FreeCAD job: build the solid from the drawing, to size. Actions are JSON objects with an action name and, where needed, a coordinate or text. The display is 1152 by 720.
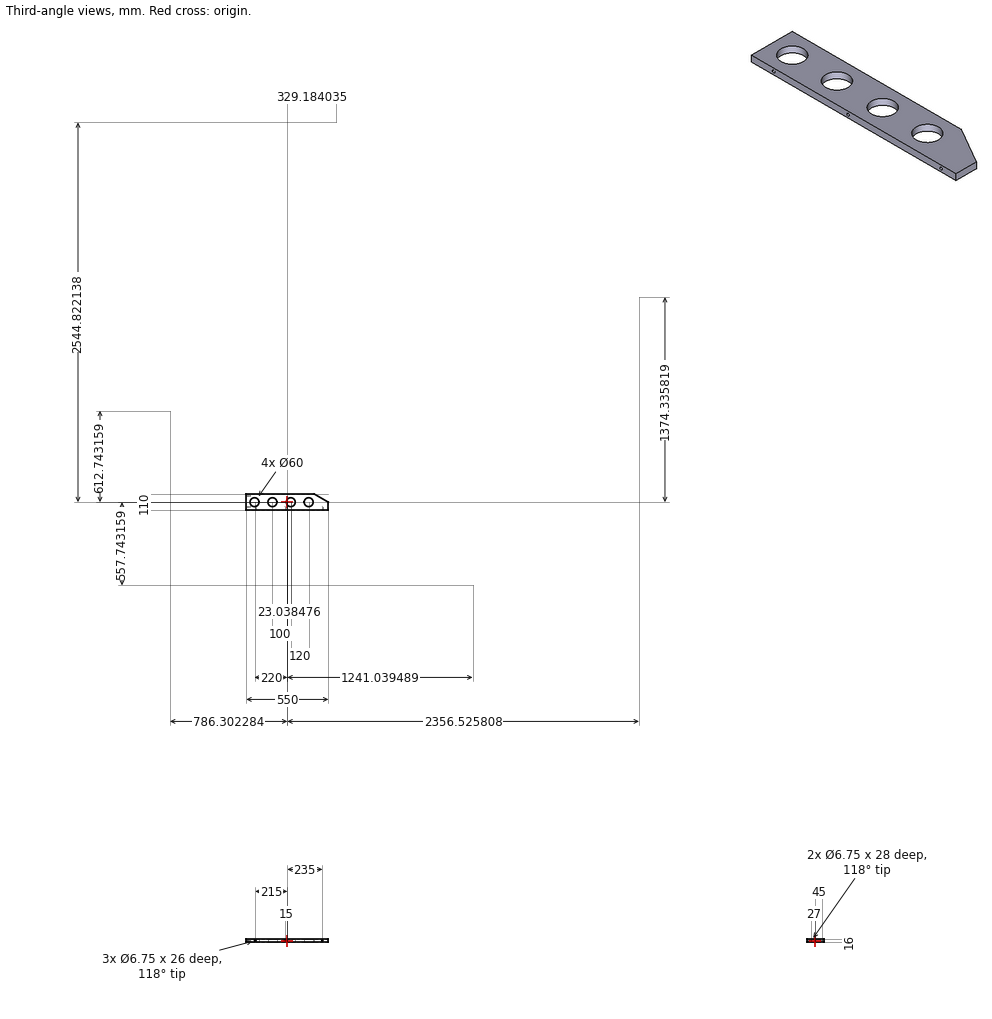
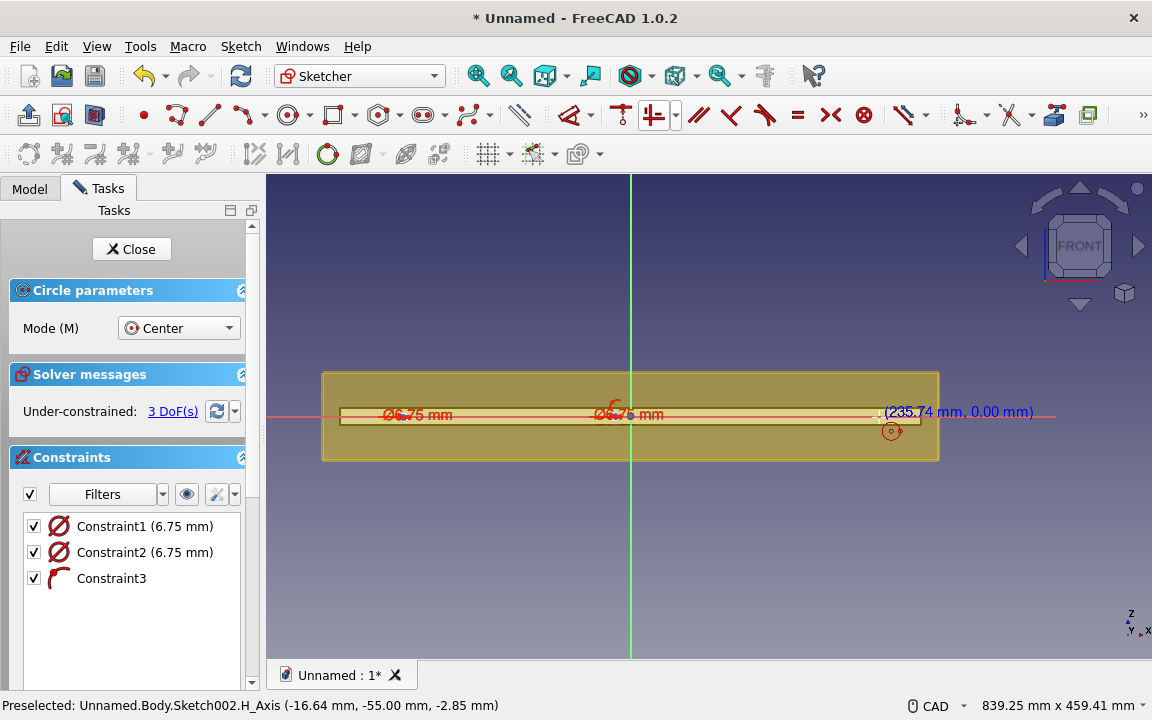
{"action": "left_click", "coordinate": [879, 417]}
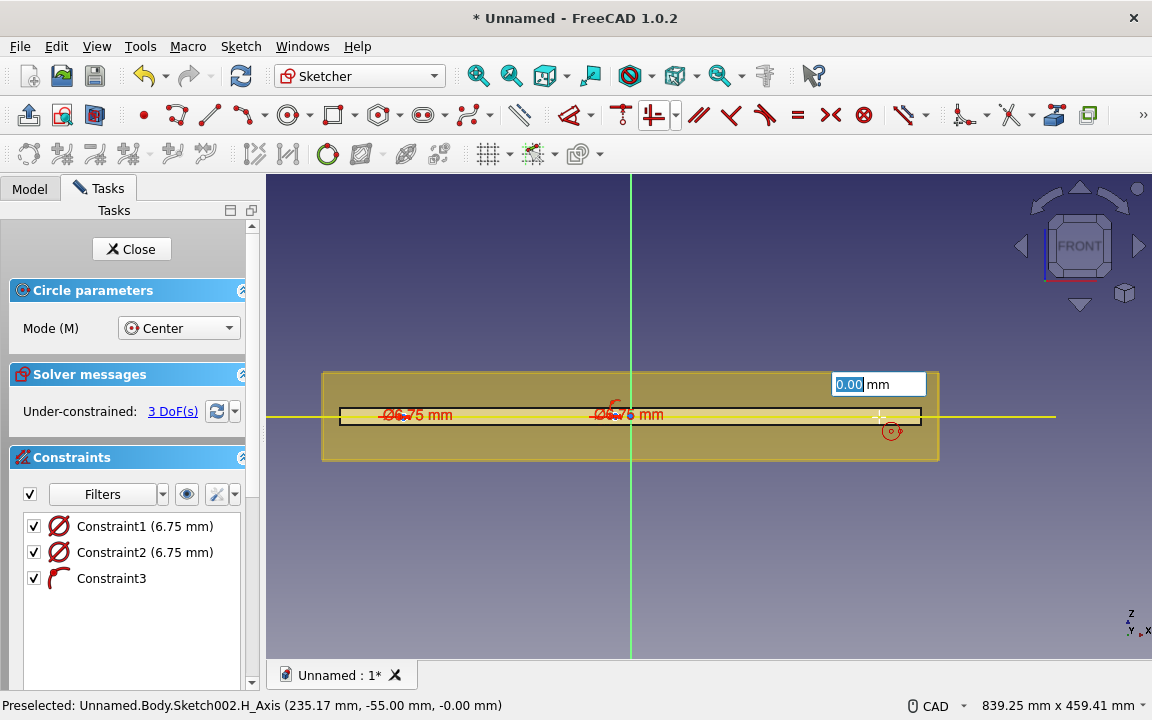
{"action": "scroll", "coordinate": [878, 420], "scroll_direction": "up", "scroll_amount": 8}
{"action": "mouse_move", "coordinate": [873, 418]}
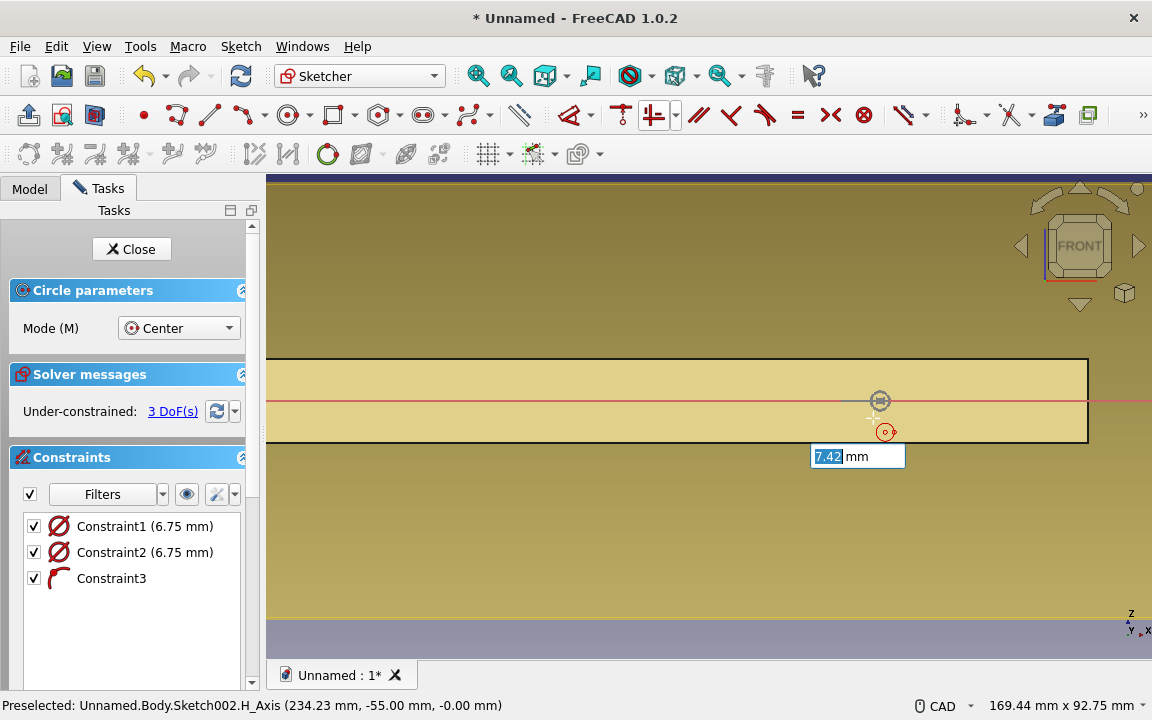
{"action": "type", "text": "6.75"}
{"action": "key", "text": "Return"}
{"action": "key", "text": "Escape"}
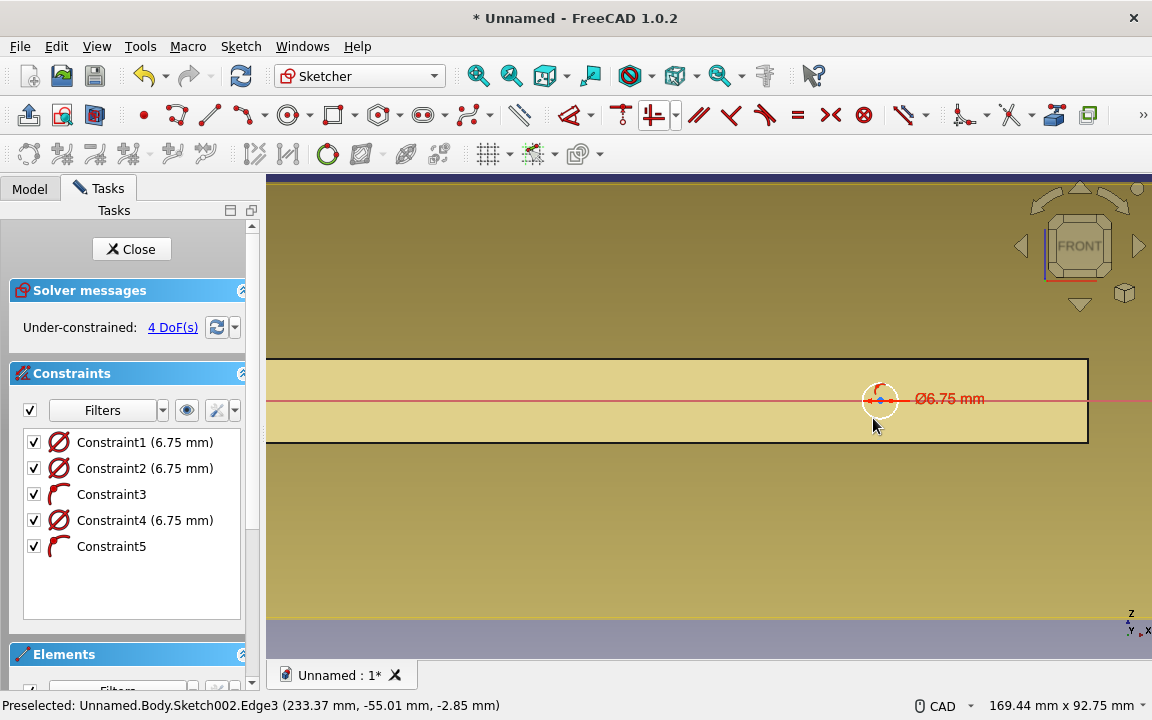
{"action": "scroll", "coordinate": [878, 420], "scroll_direction": "down", "scroll_amount": 8}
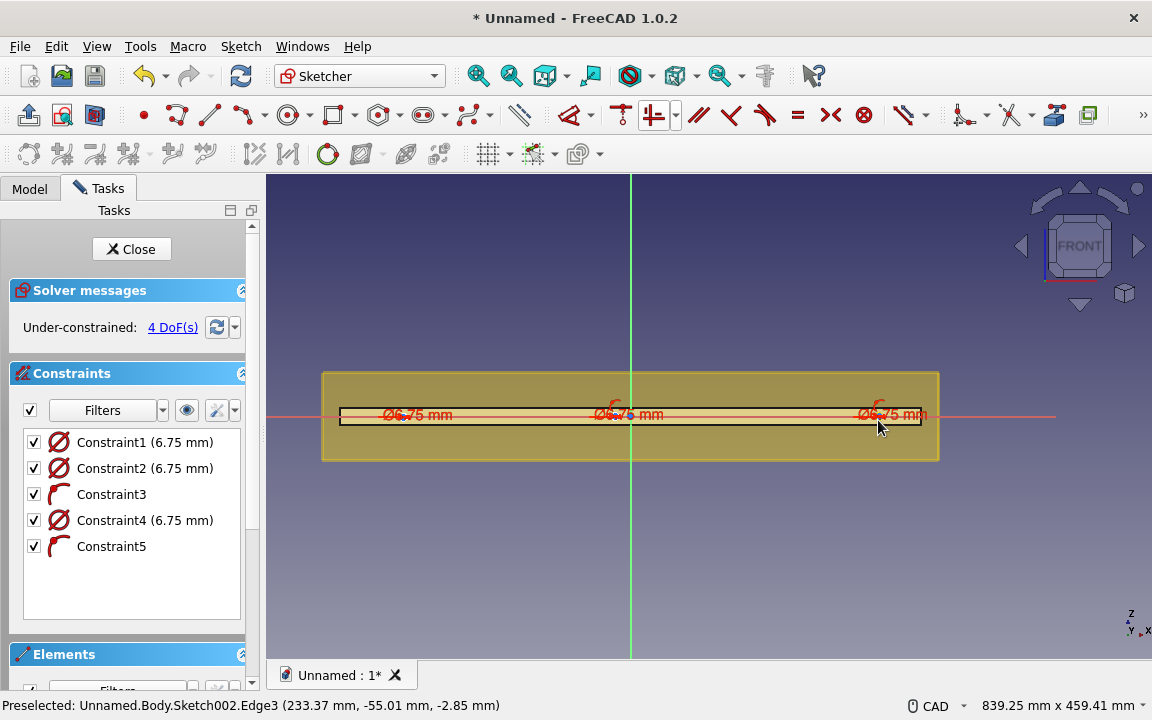
{"action": "left_click", "coordinate": [404, 417]}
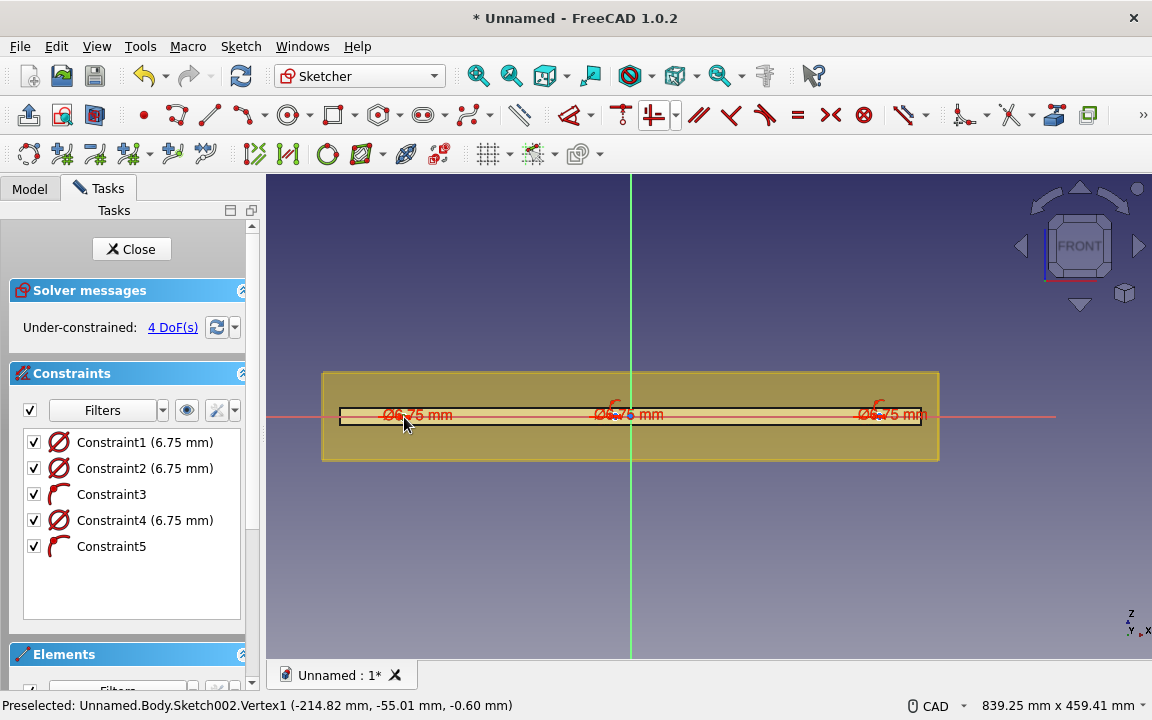
{"action": "left_click", "coordinate": [344, 417]}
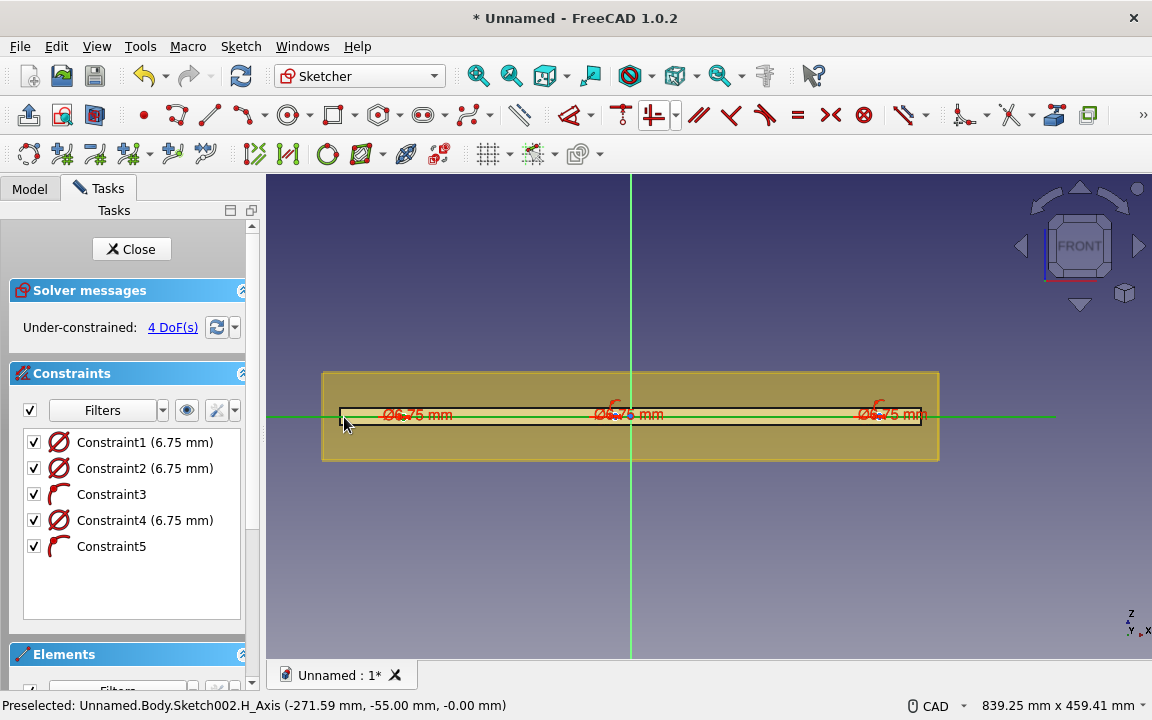
{"action": "left_click", "coordinate": [621, 116]}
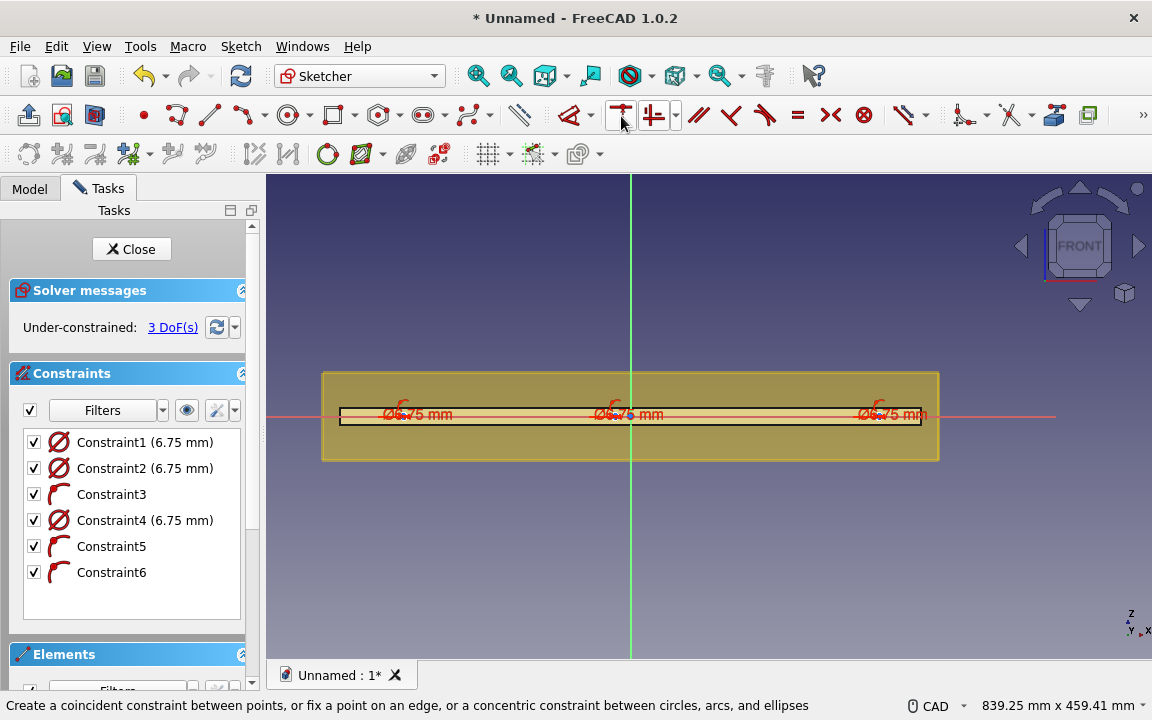
{"action": "key", "text": "d"}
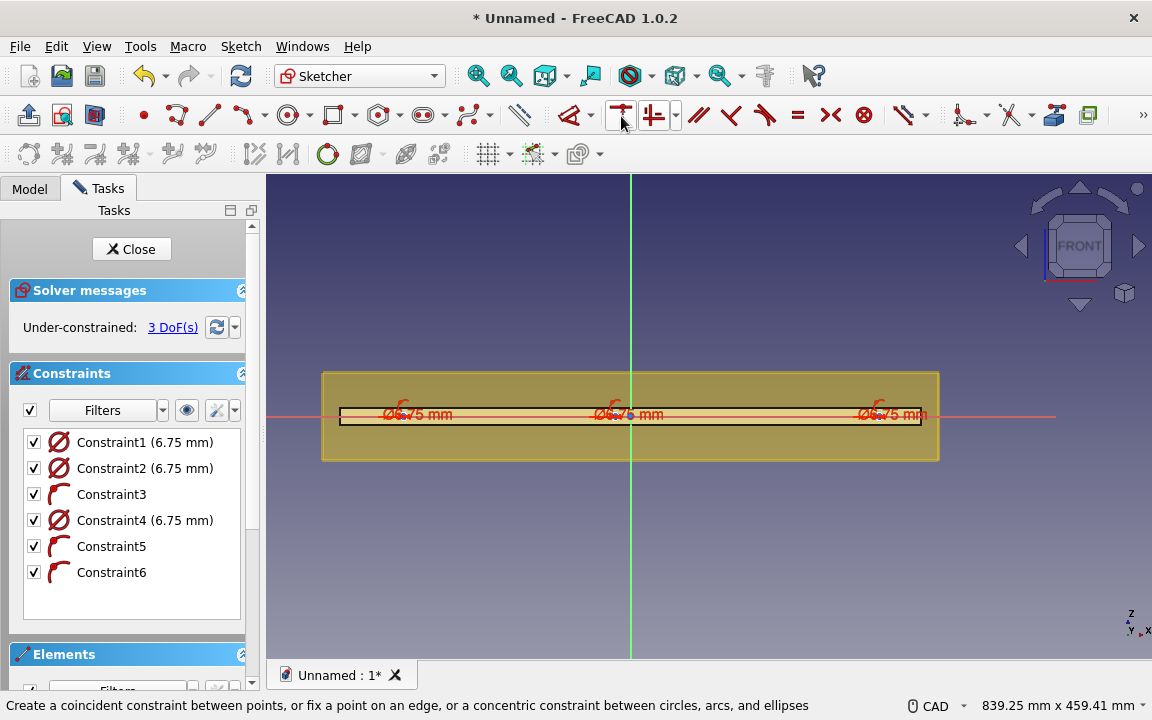
{"action": "scroll", "coordinate": [615, 417], "scroll_direction": "up", "scroll_amount": 5}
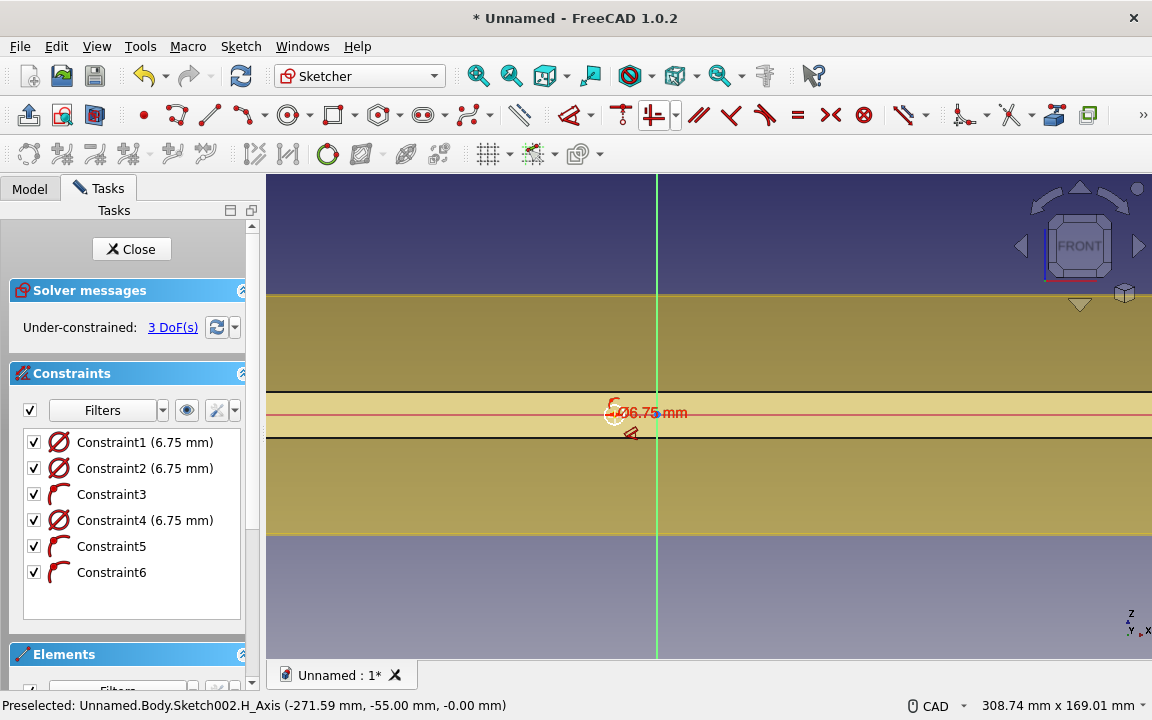
{"action": "left_click", "coordinate": [615, 415]}
{"action": "left_click", "coordinate": [636, 449]}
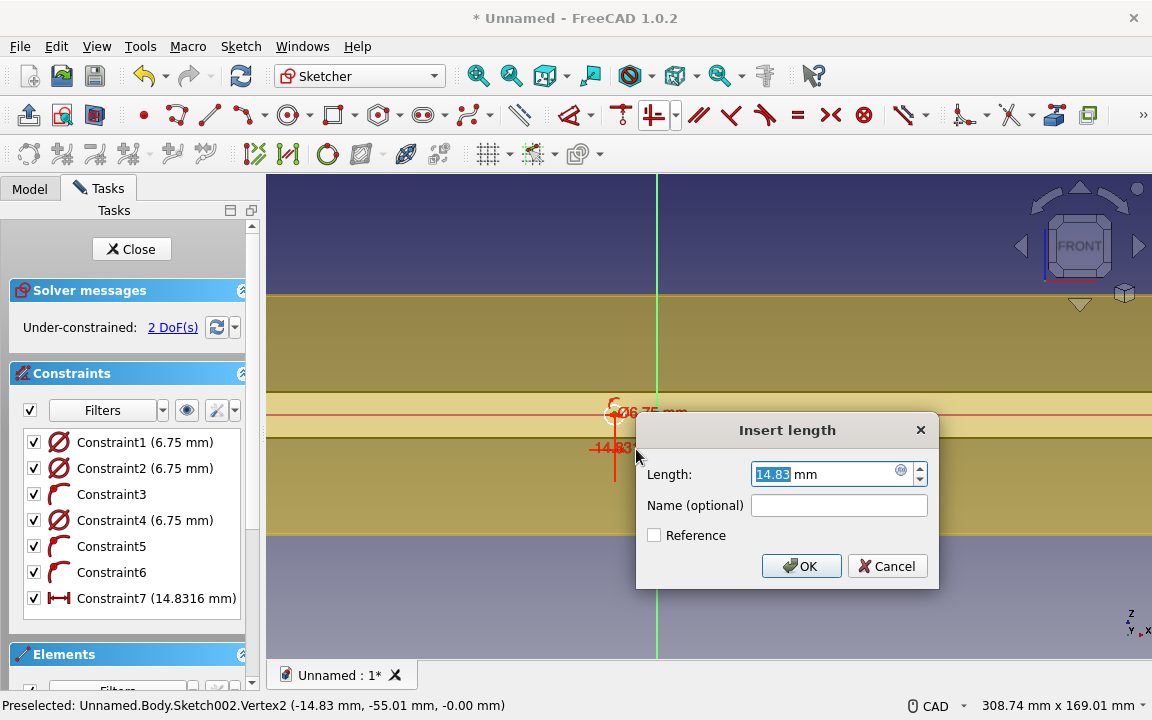
{"action": "type", "text": "15"}
{"action": "key", "text": "Return"}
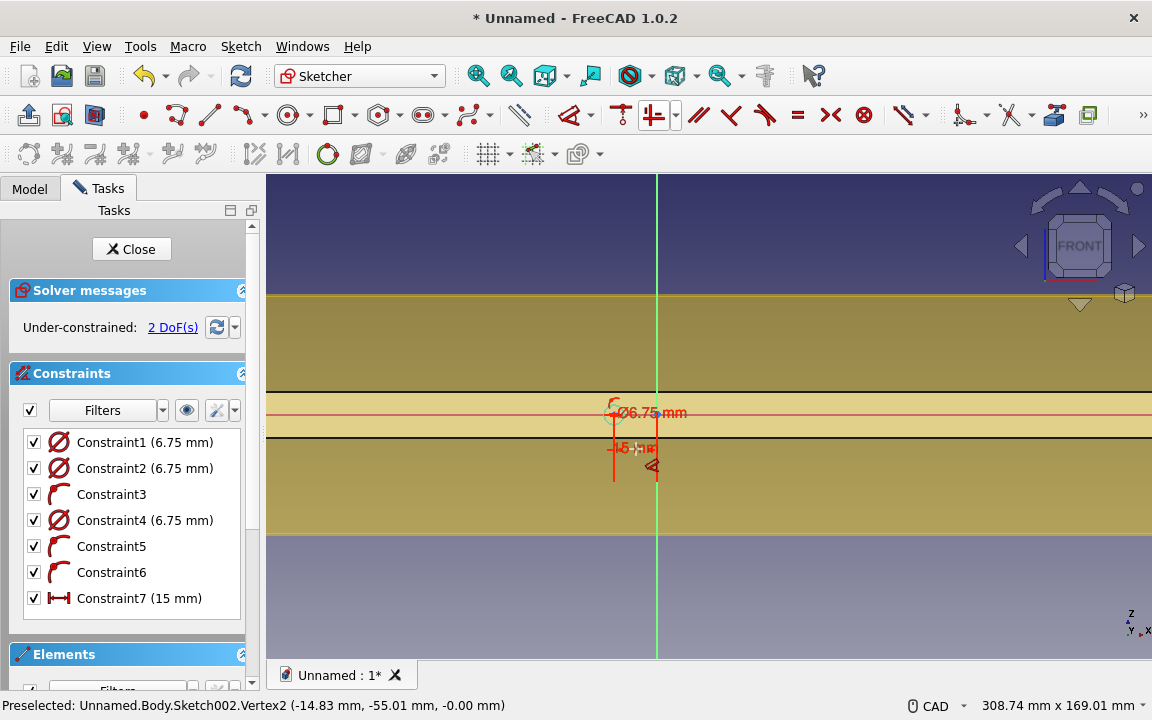
{"action": "scroll", "coordinate": [614, 417], "scroll_direction": "down", "scroll_amount": 5}